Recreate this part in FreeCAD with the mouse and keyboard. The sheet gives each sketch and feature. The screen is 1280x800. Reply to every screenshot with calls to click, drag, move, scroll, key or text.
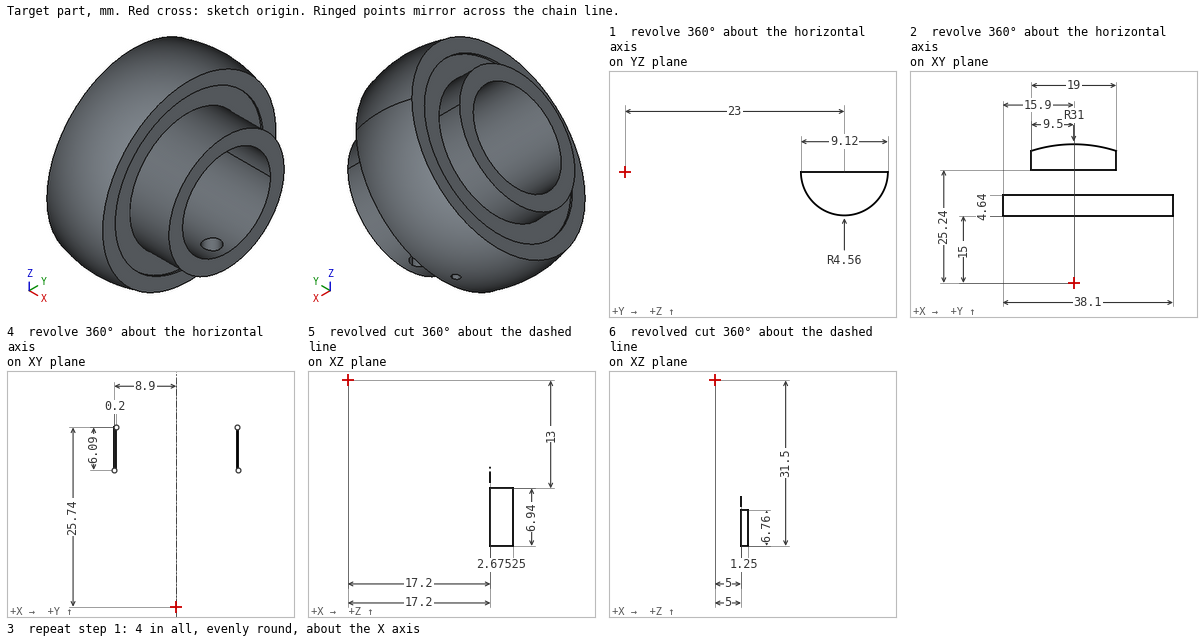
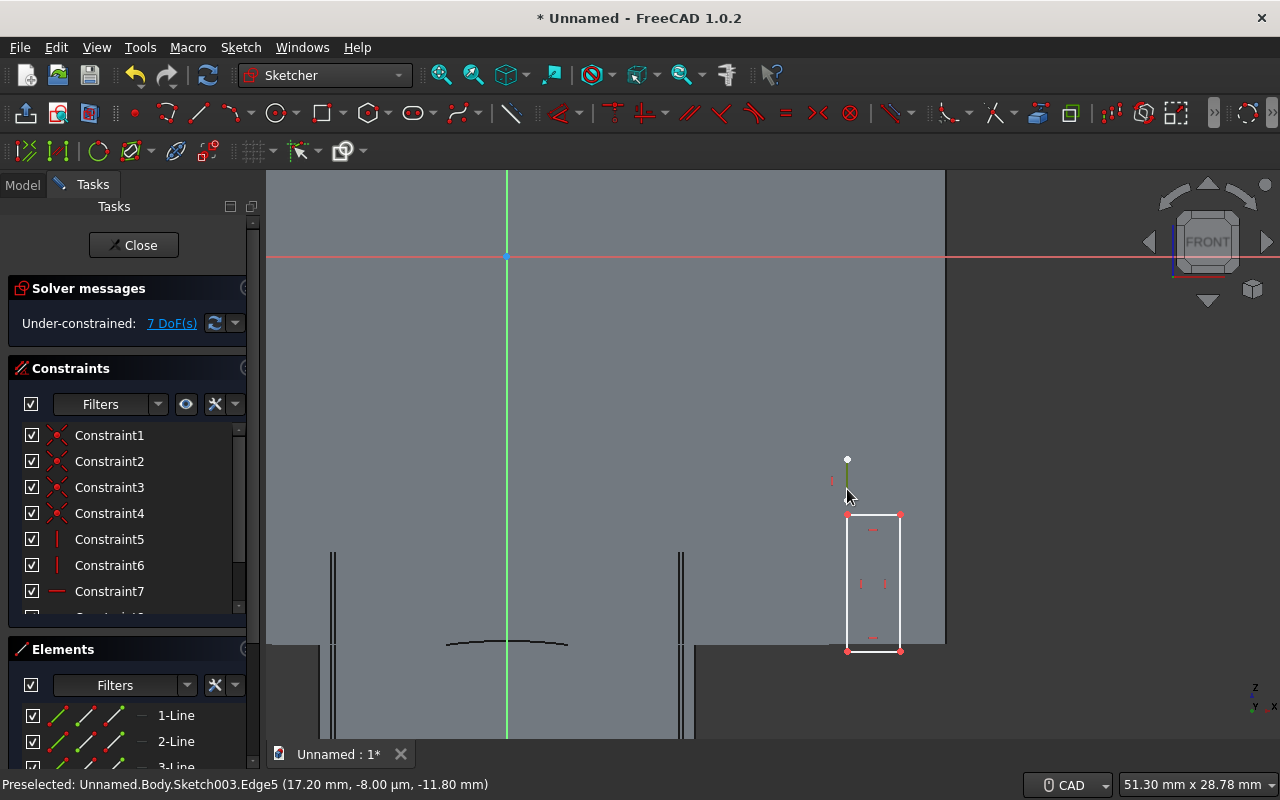
click(512, 114)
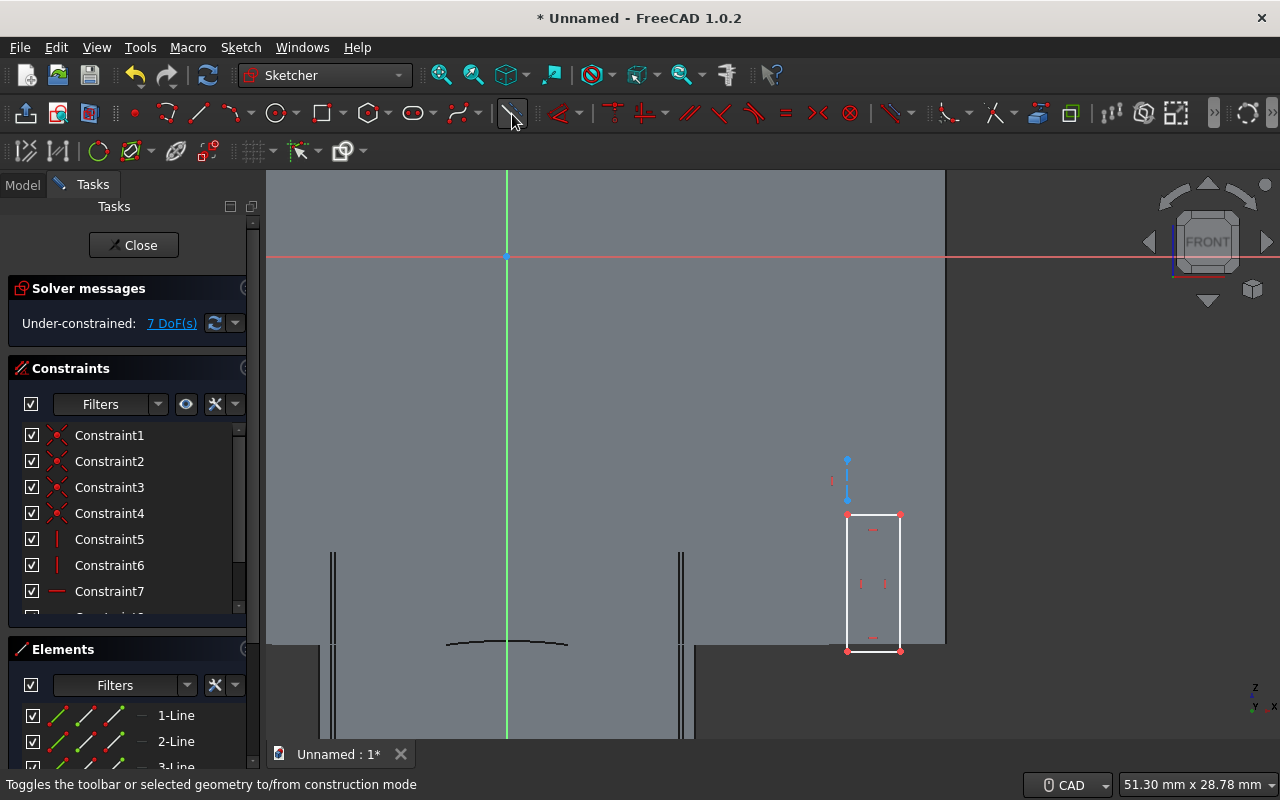
click(558, 114)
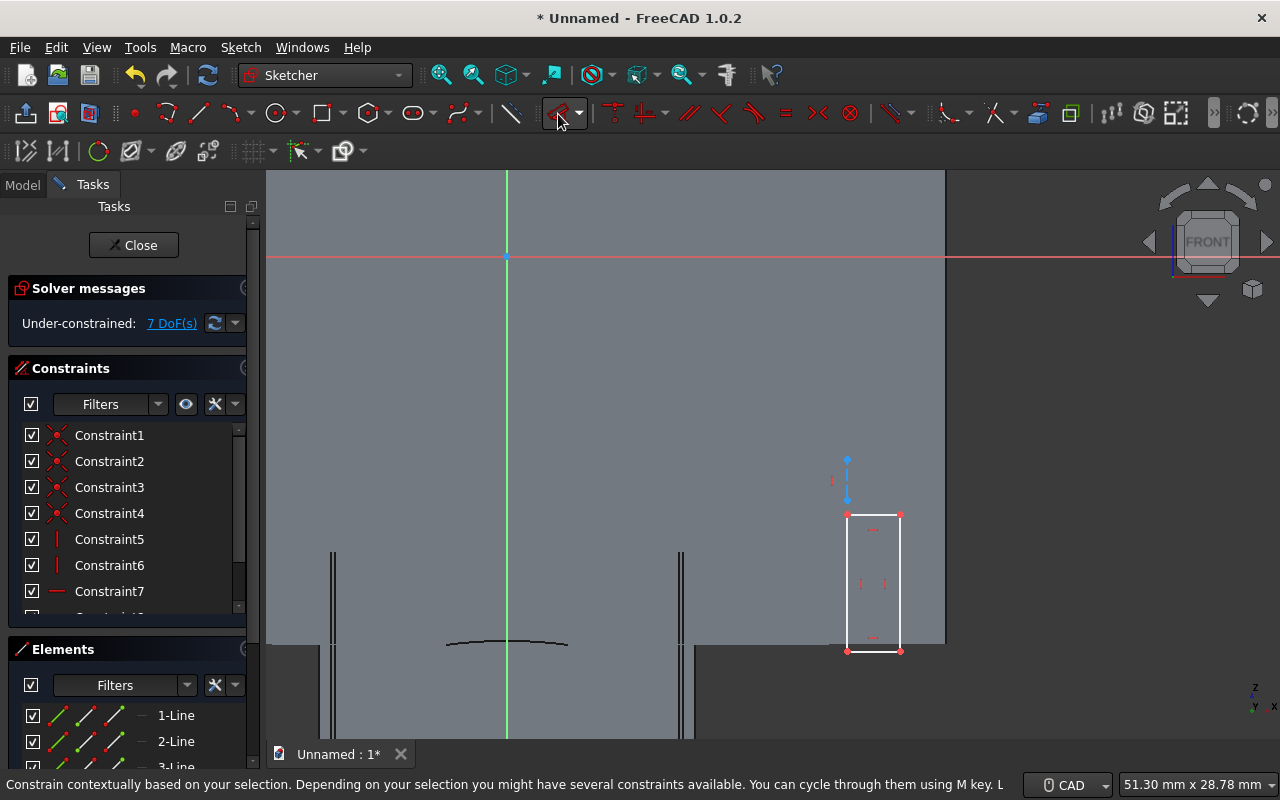
click(847, 515)
click(473, 386)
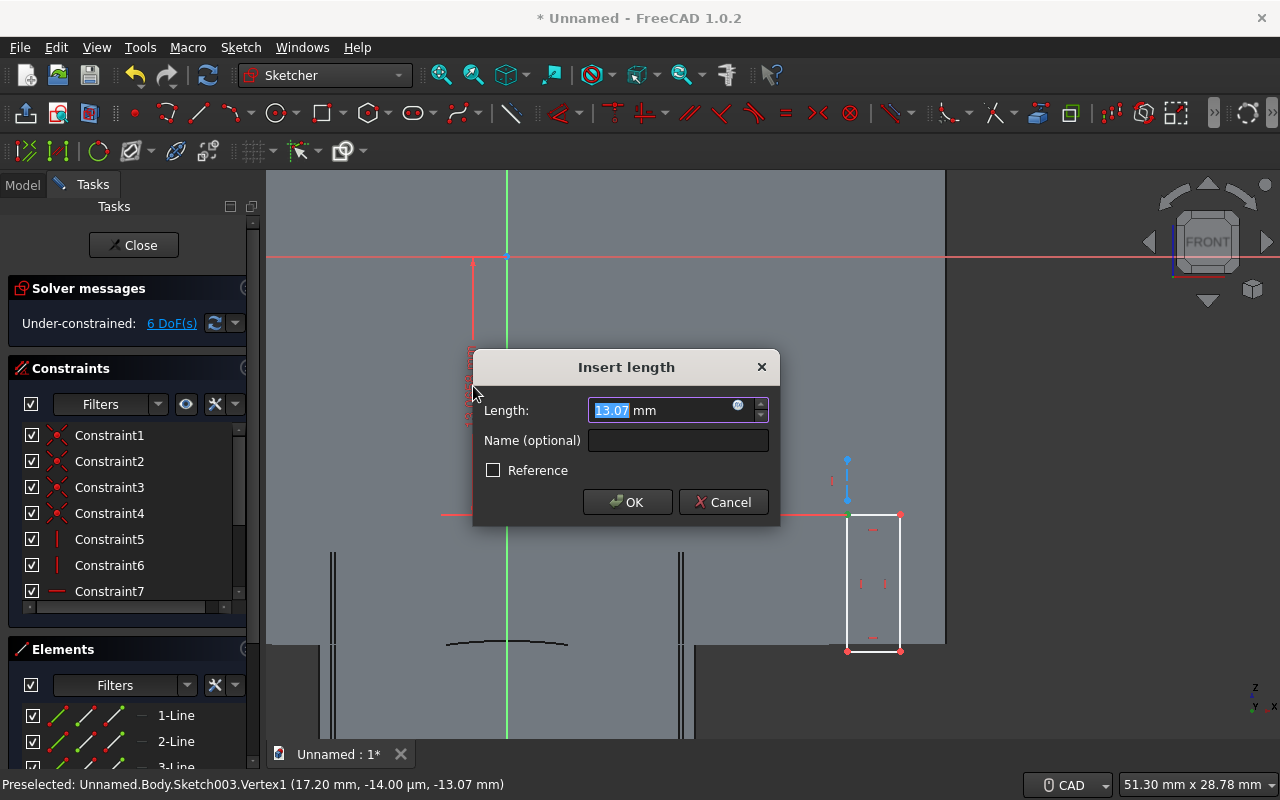
text(13)
key(Return)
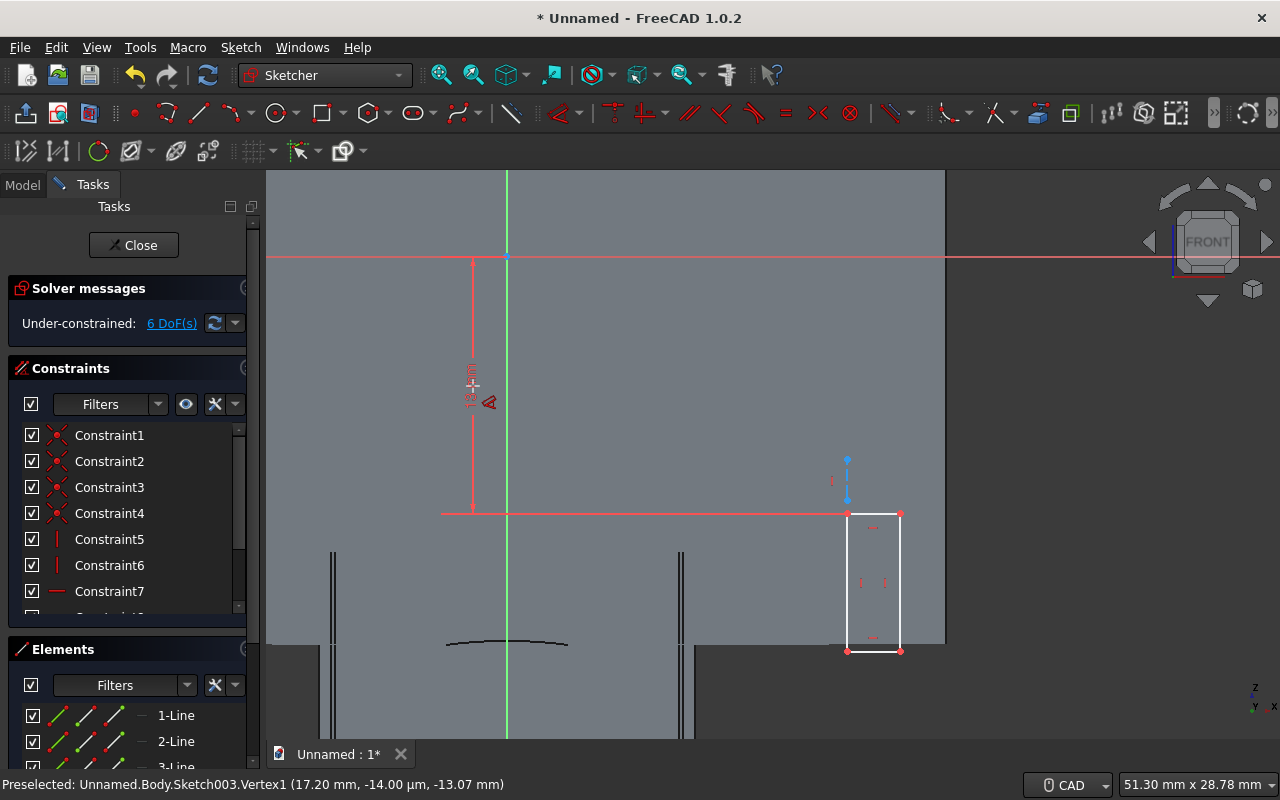
click(847, 555)
click(881, 583)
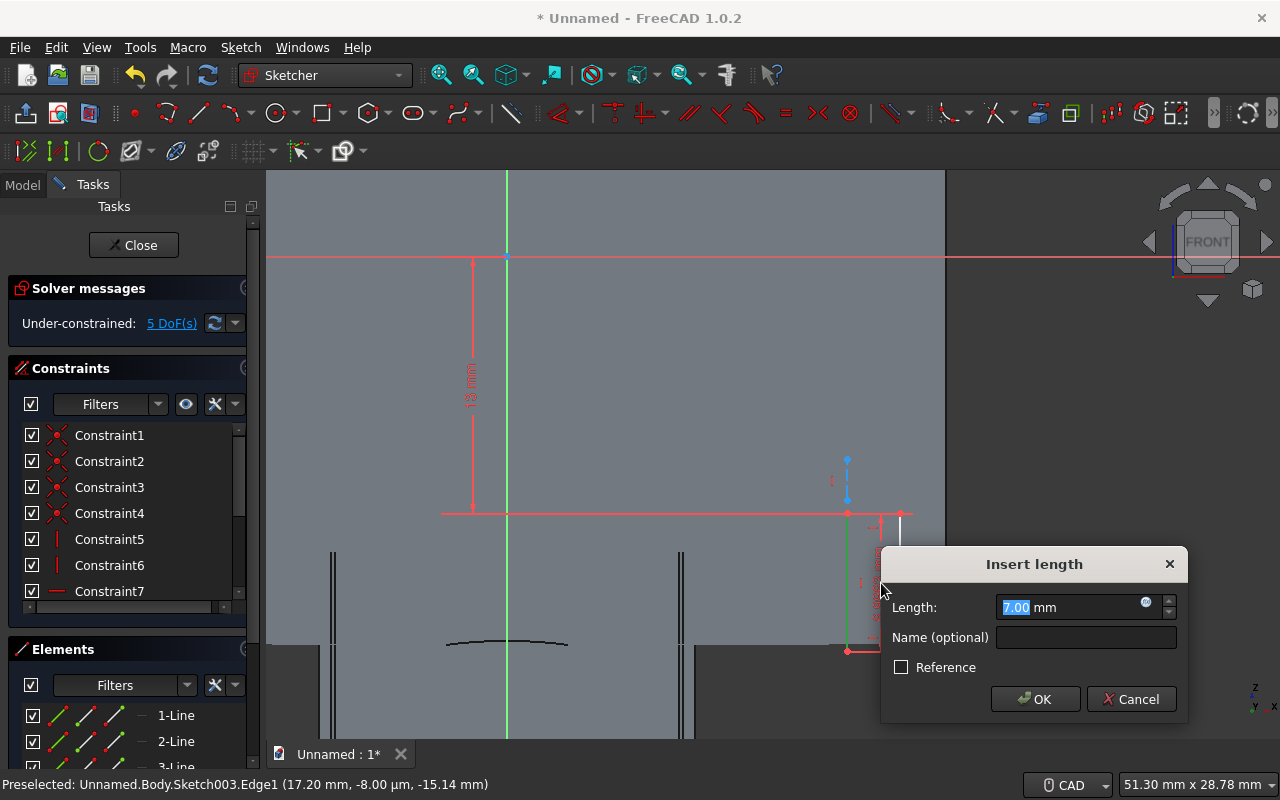
text(6.94)
key(Return)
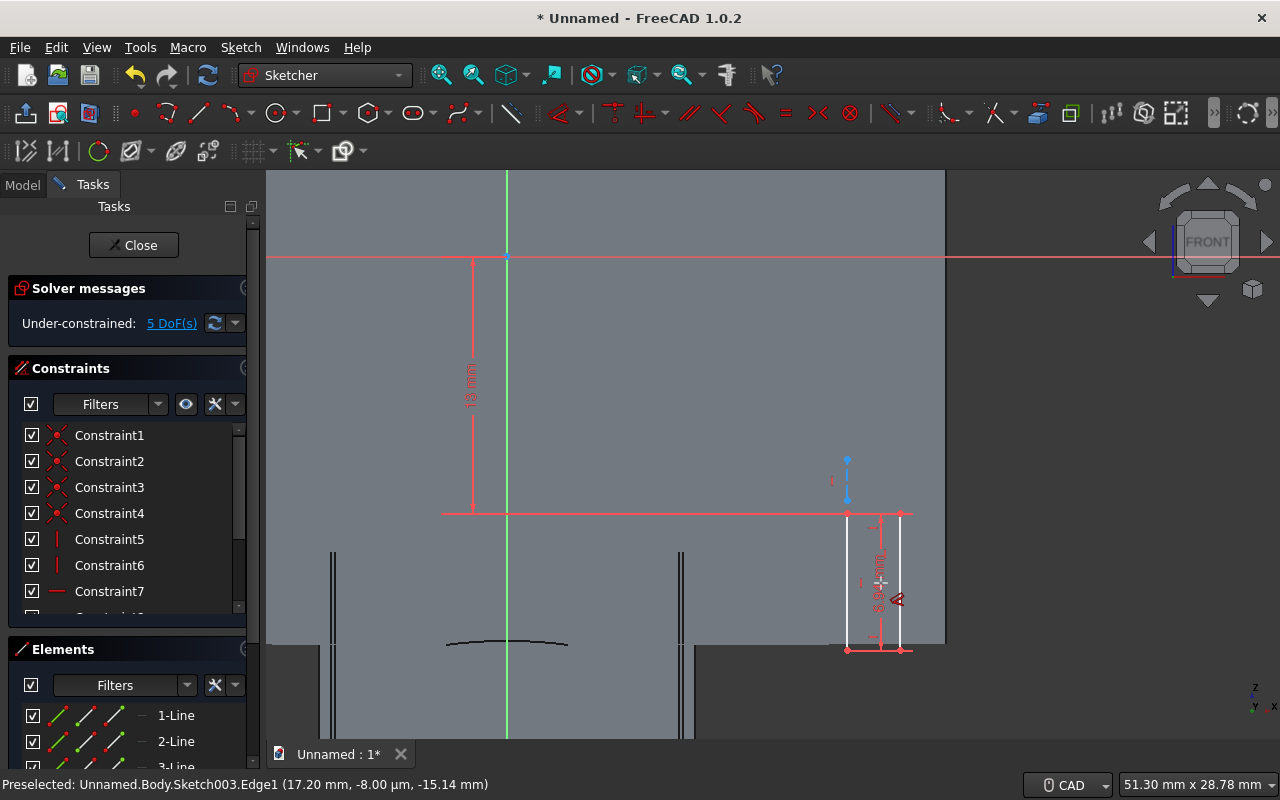
click(847, 514)
click(677, 223)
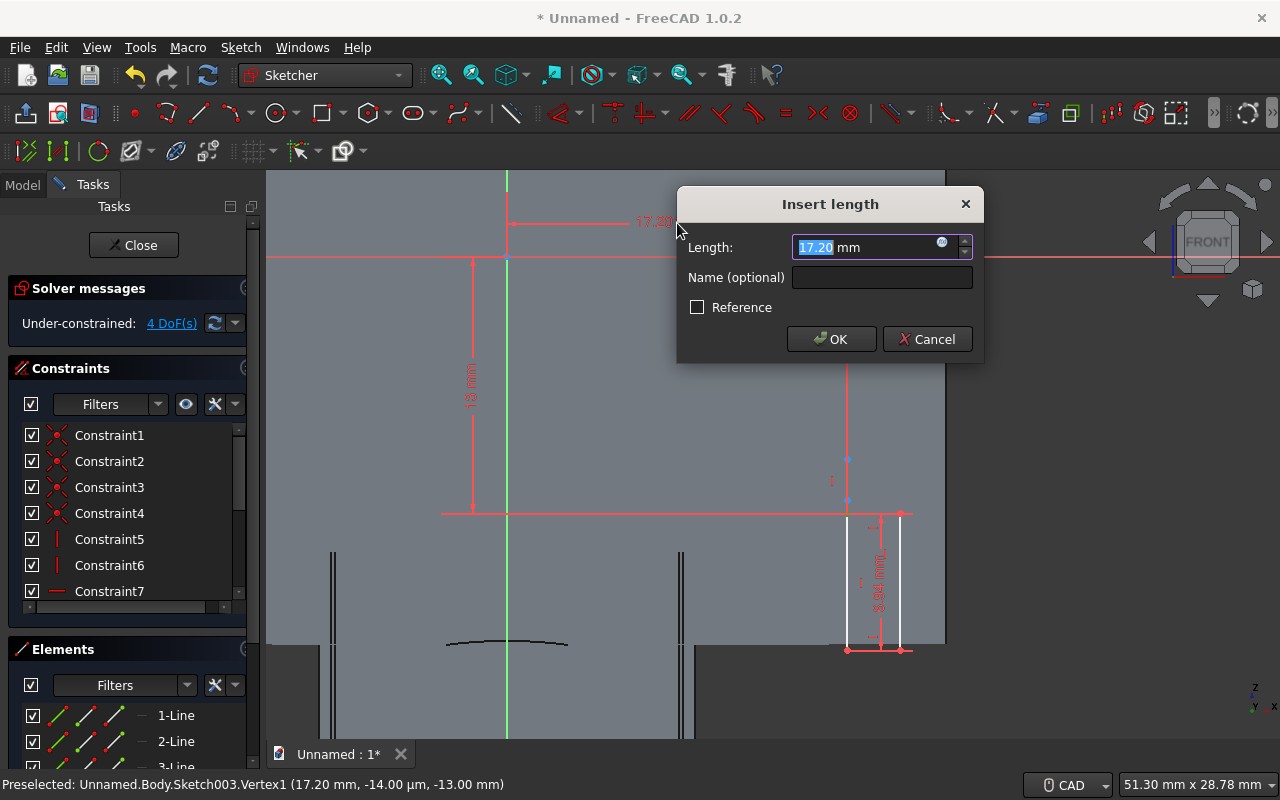
text(17.2)
key(Return)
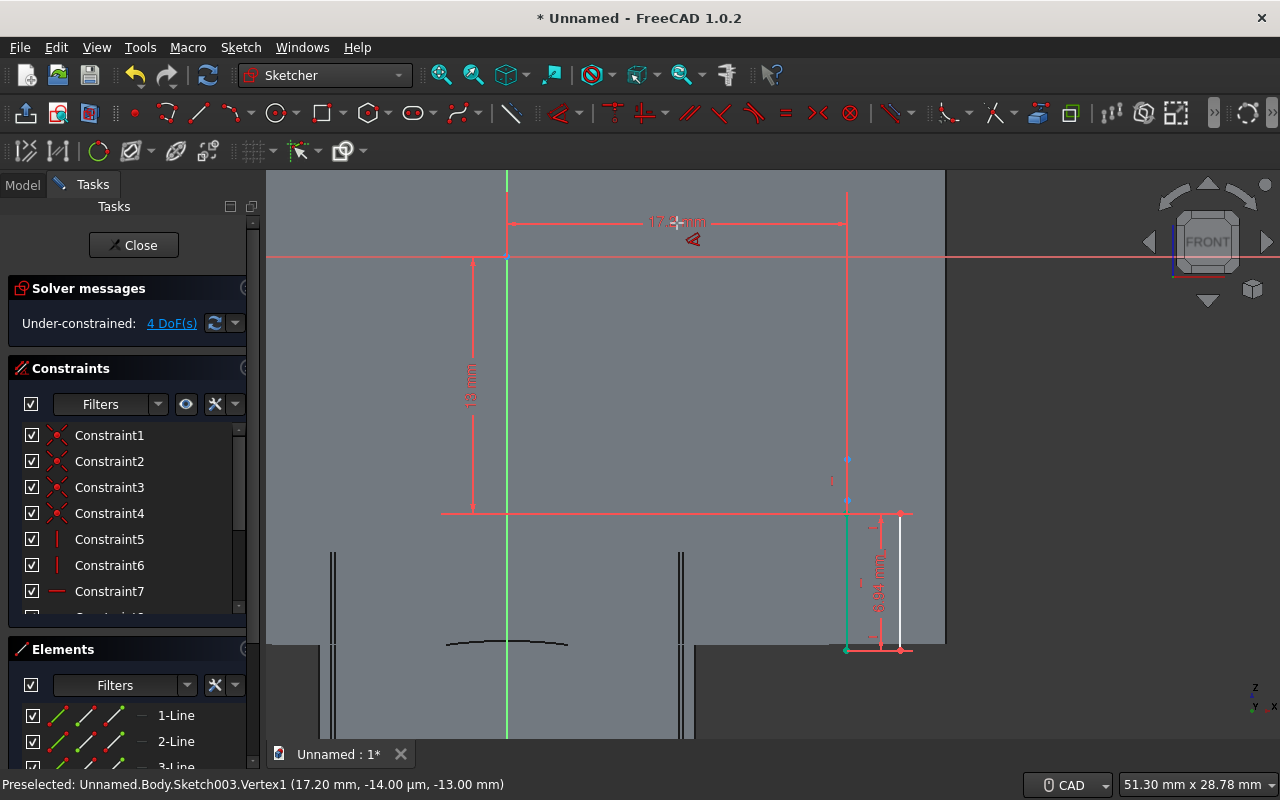
click(847, 501)
click(599, 223)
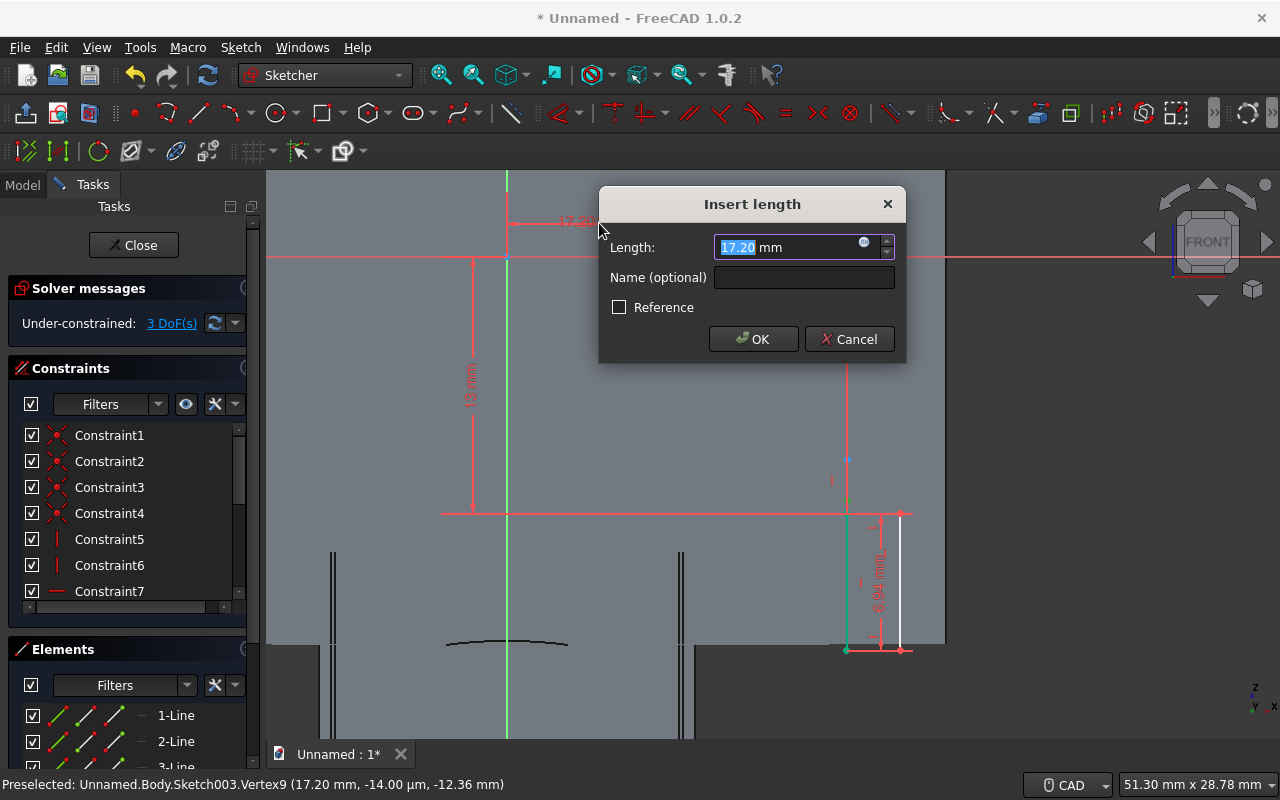
text(17.2)
key(Return)